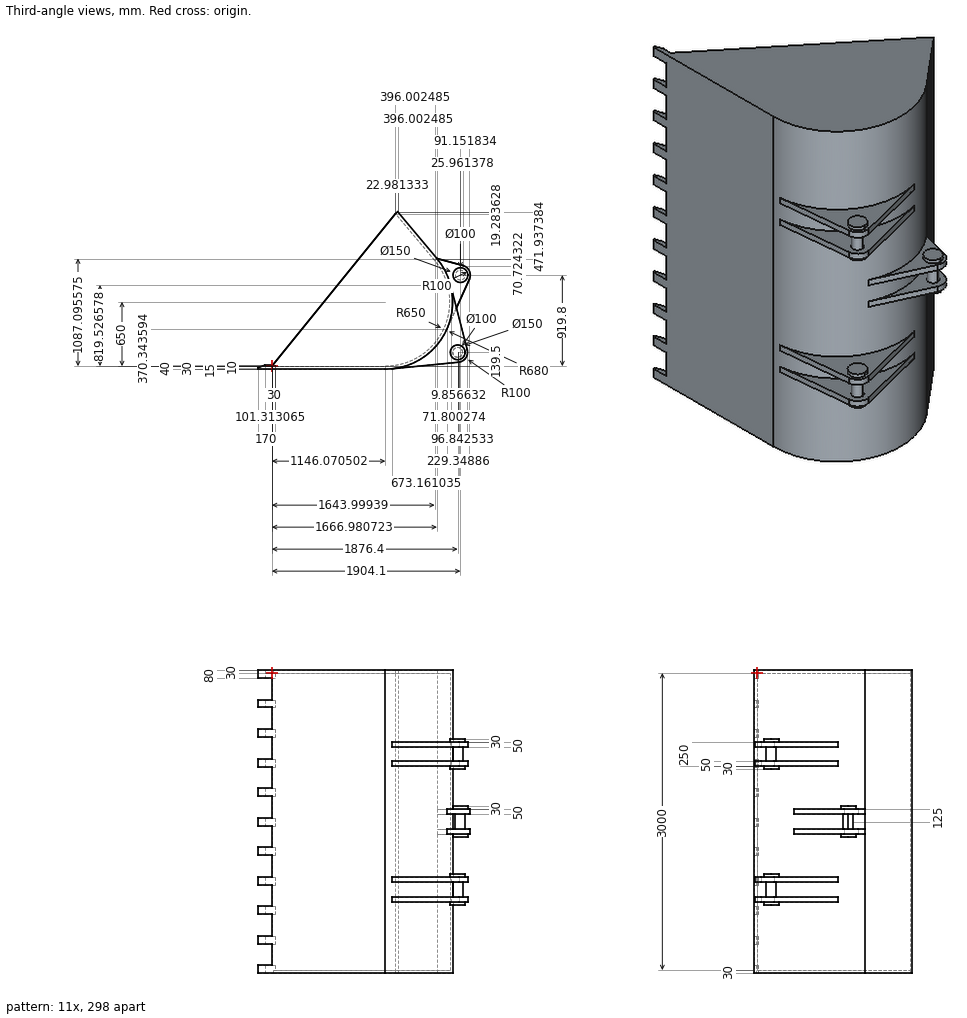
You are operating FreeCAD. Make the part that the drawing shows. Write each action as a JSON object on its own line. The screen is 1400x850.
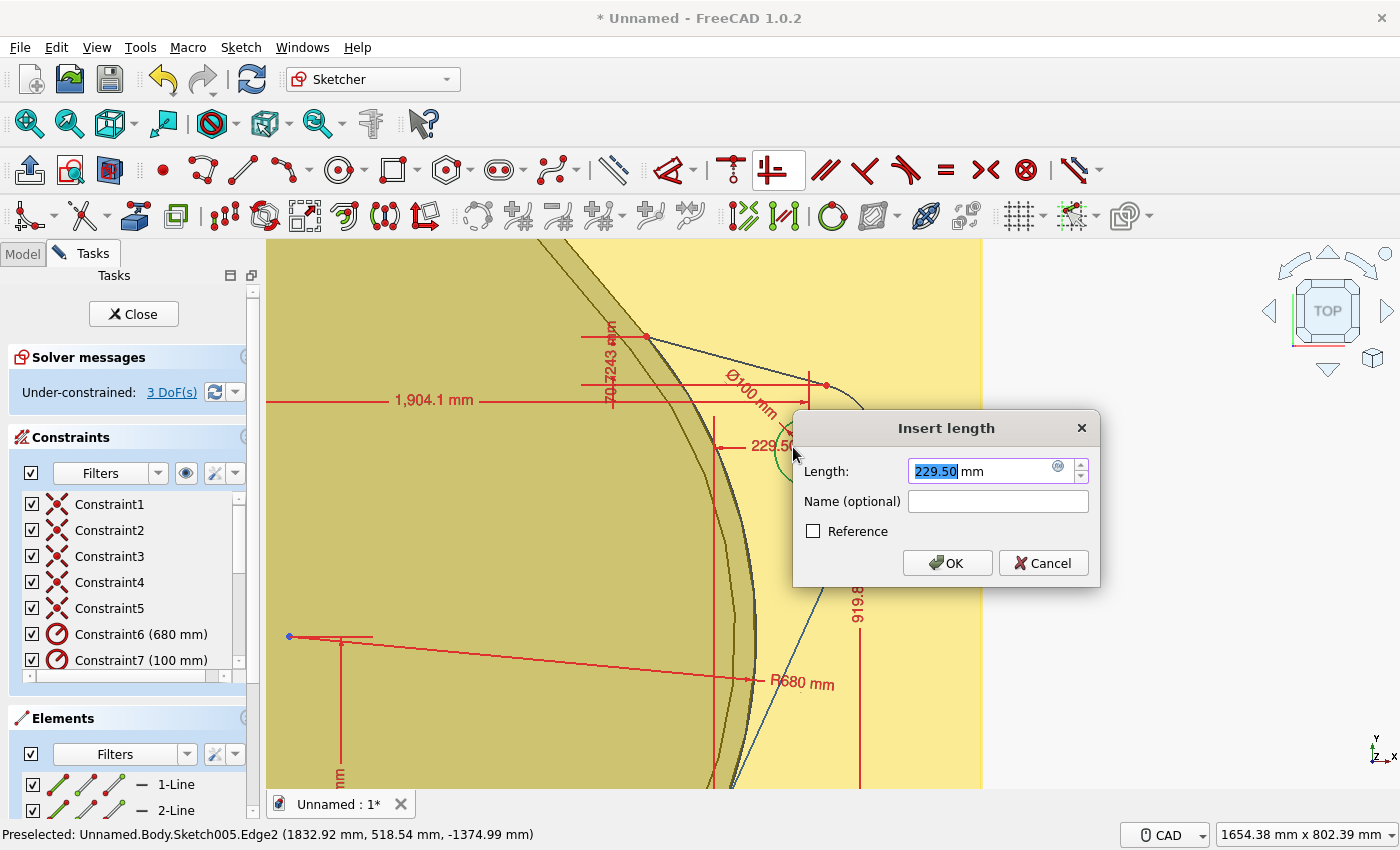
{"action": "type", "text": "229.34886"}
{"action": "key", "text": "Return"}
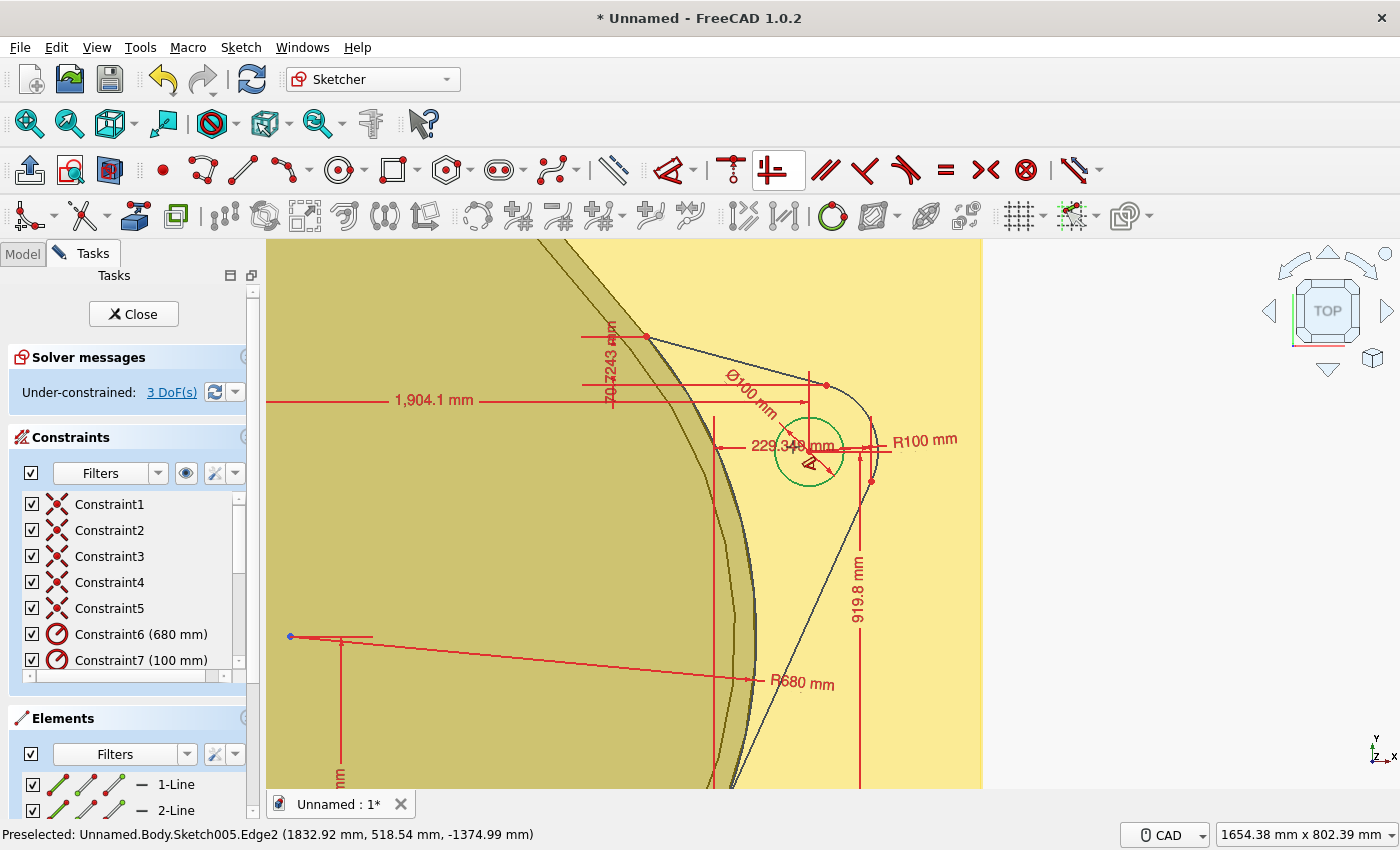
{"action": "scroll", "coordinate": [826, 385], "scroll_direction": "up", "scroll_amount": 5}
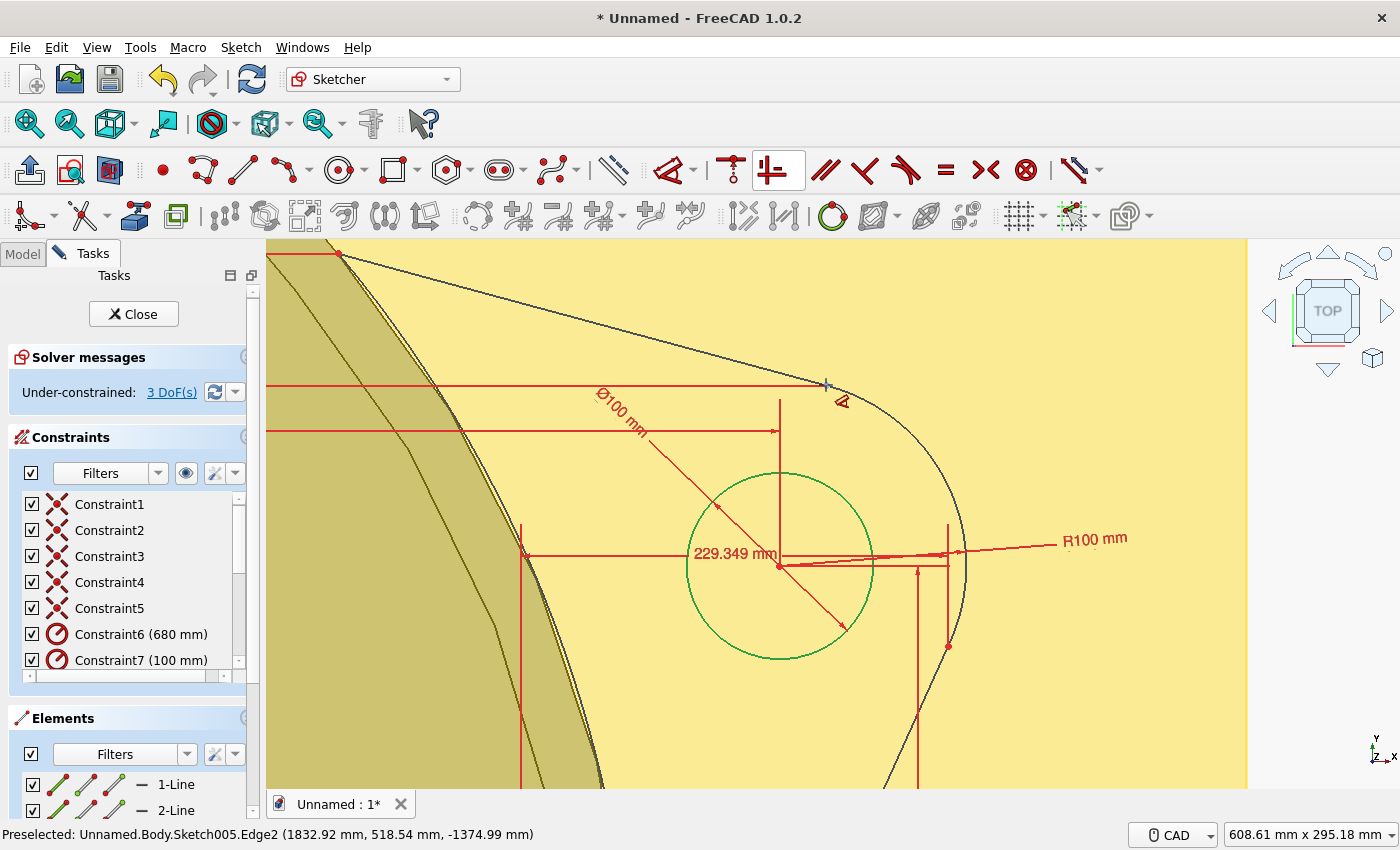
{"action": "left_click", "coordinate": [826, 386]}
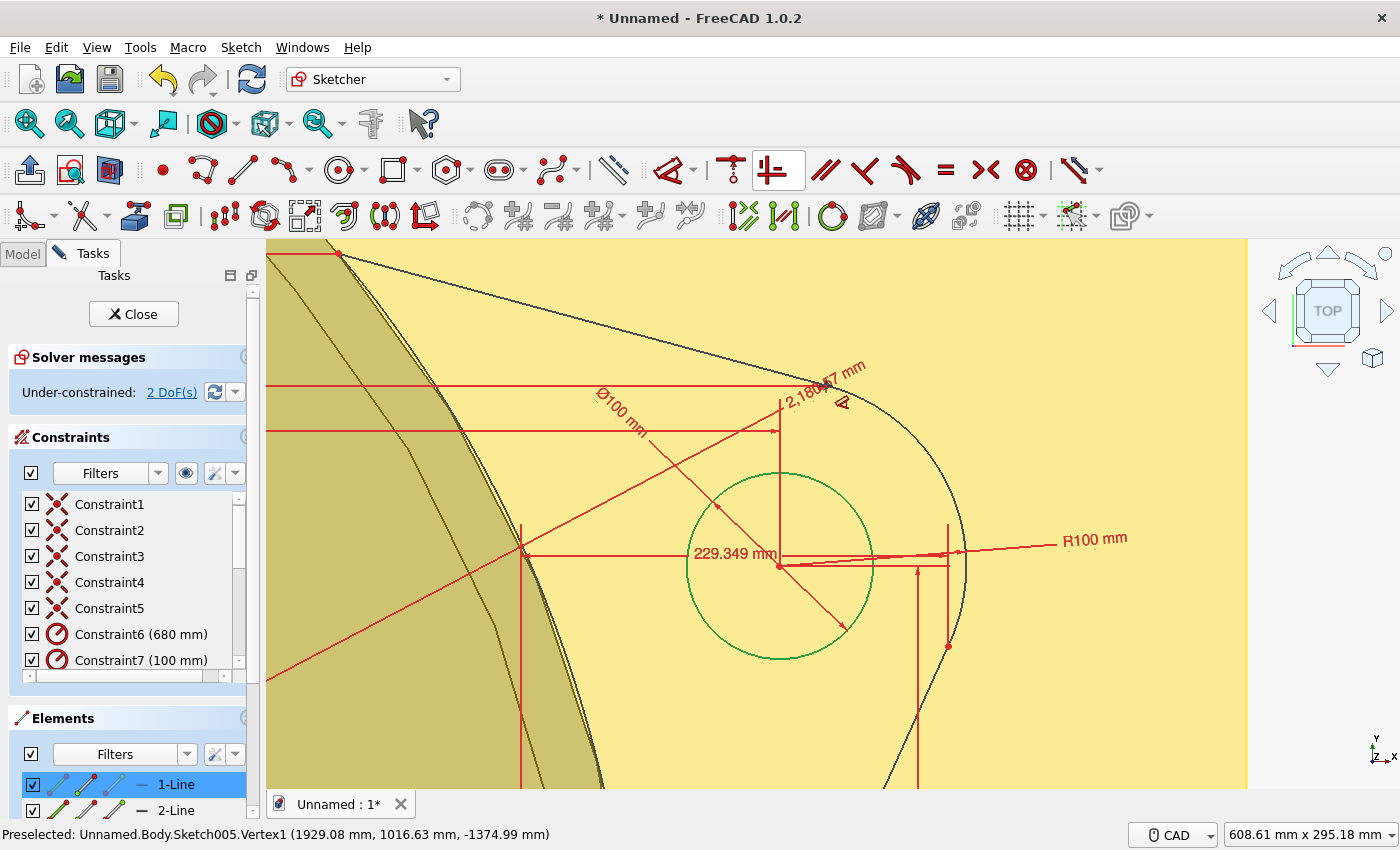
{"action": "left_click", "coordinate": [780, 566]}
{"action": "left_click", "coordinate": [803, 352]}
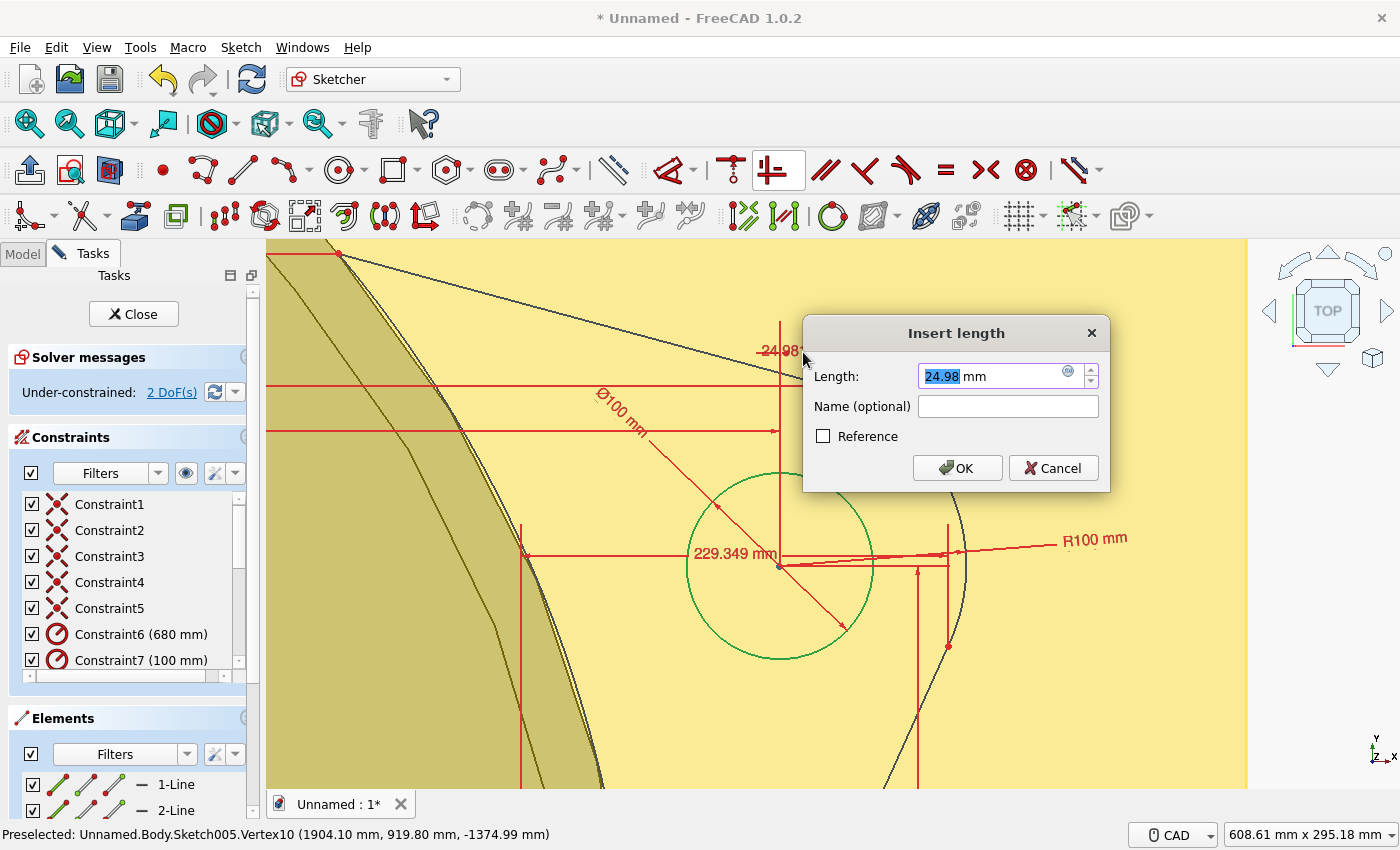
{"action": "type", "text": "25.961378"}
{"action": "key", "text": "Return"}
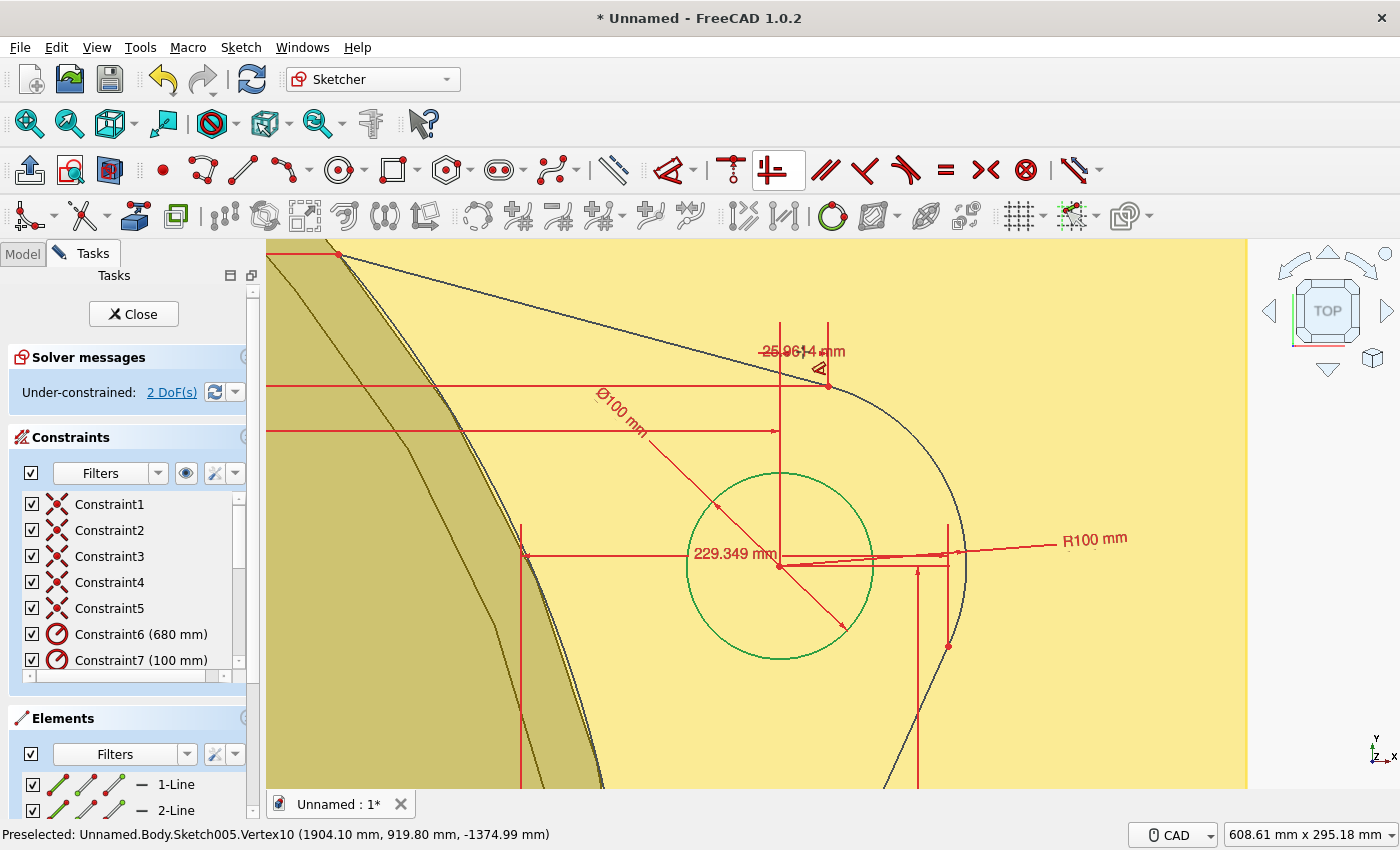
{"action": "scroll", "coordinate": [804, 380], "scroll_direction": "down", "scroll_amount": 7}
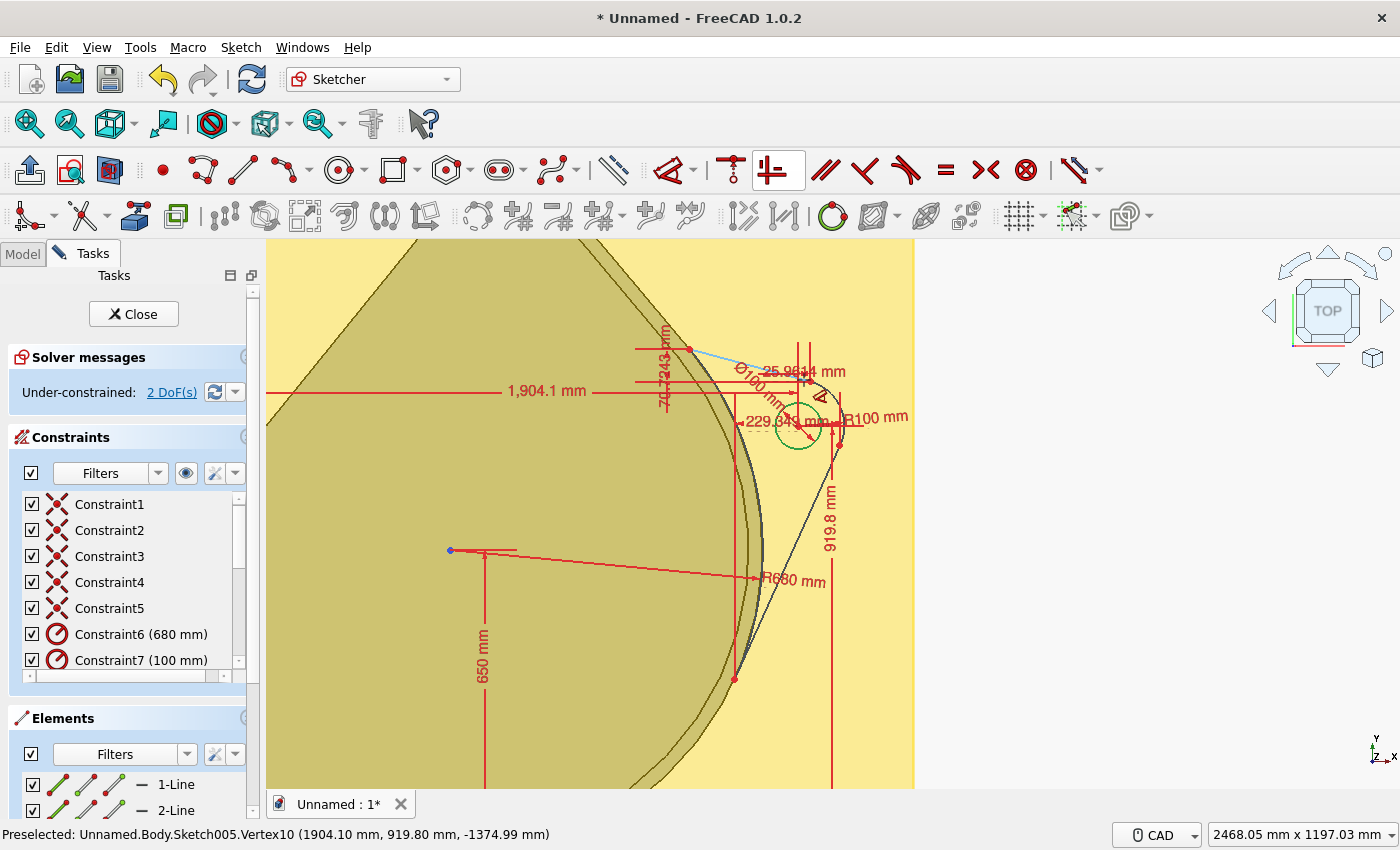
{"action": "left_click", "coordinate": [840, 446]}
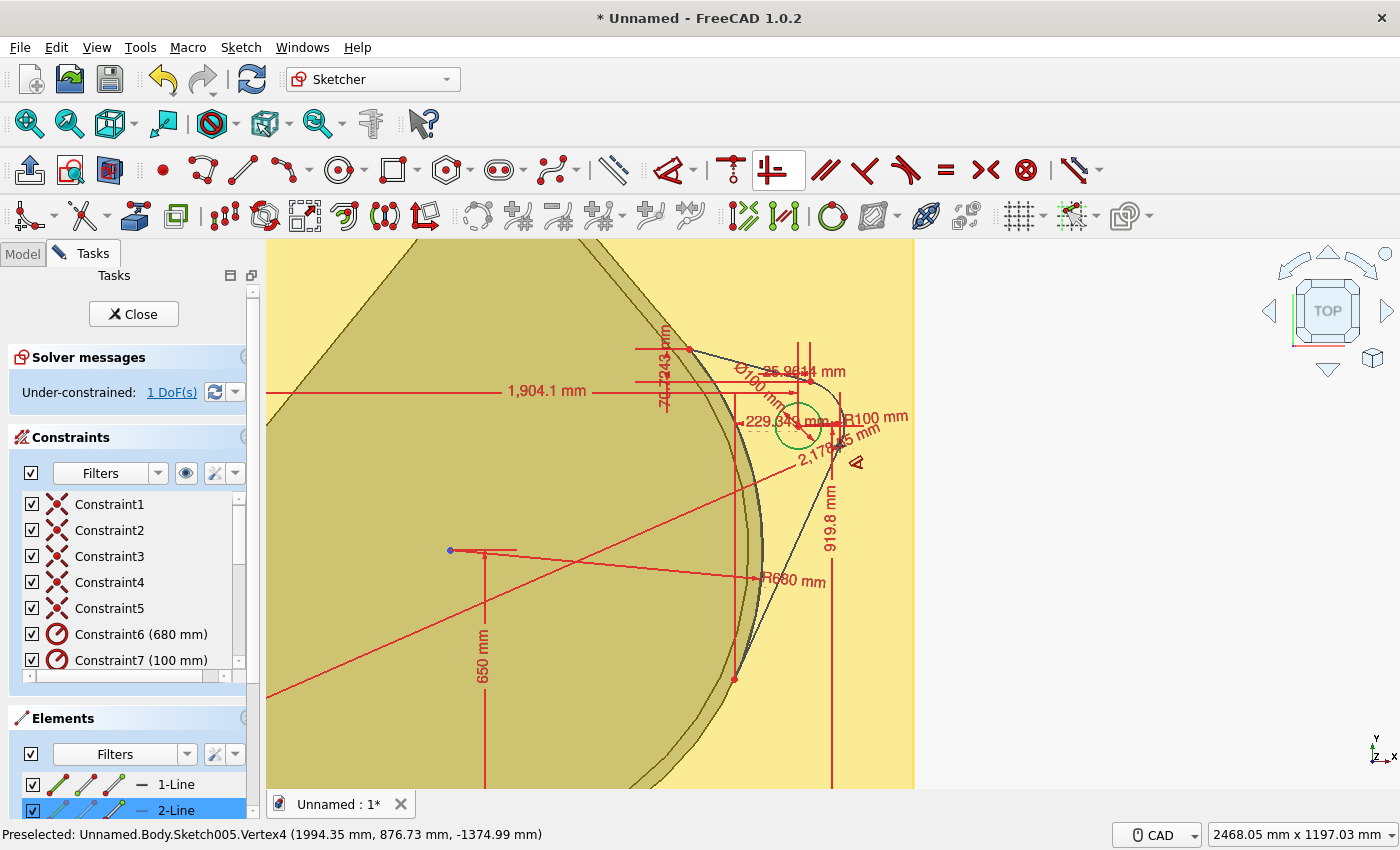
{"action": "left_click", "coordinate": [798, 426]}
{"action": "left_click", "coordinate": [810, 480]}